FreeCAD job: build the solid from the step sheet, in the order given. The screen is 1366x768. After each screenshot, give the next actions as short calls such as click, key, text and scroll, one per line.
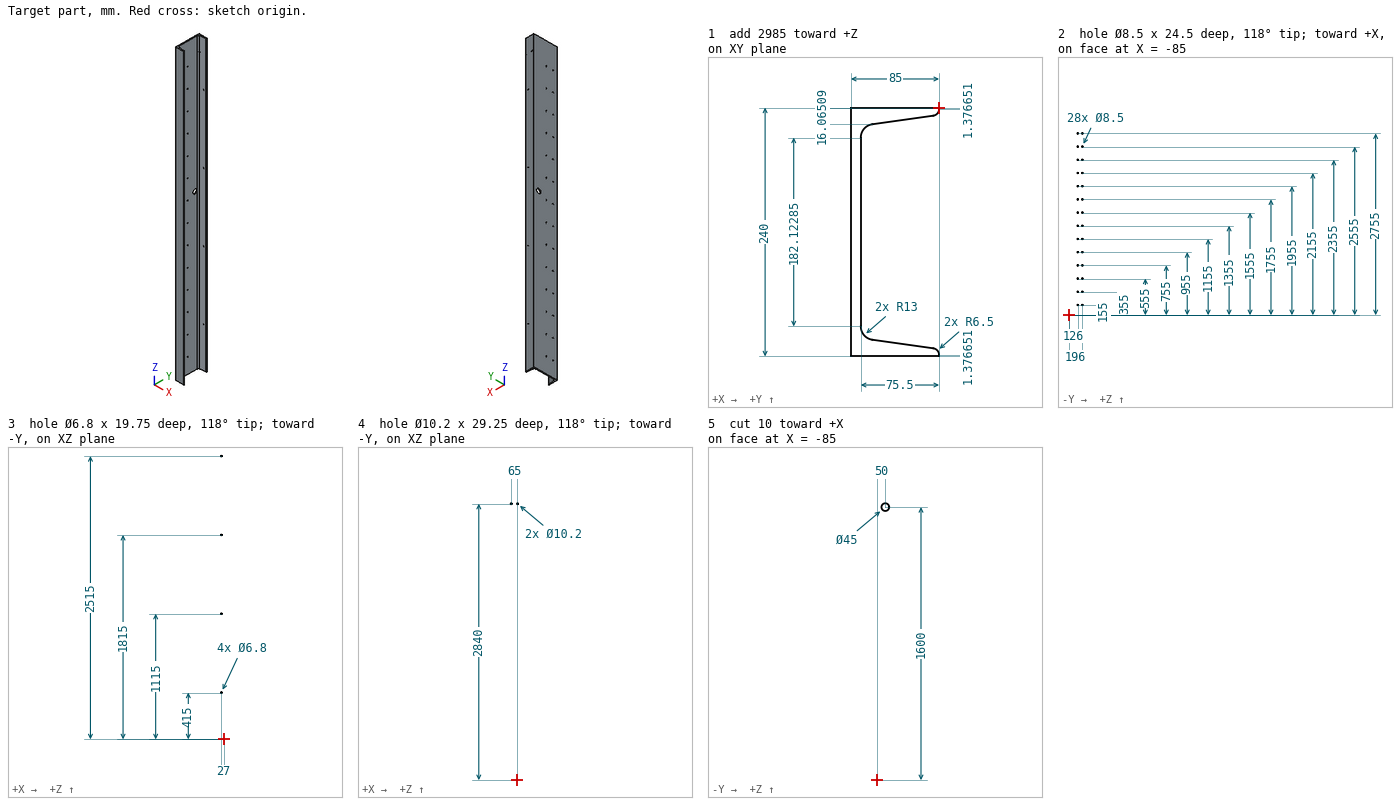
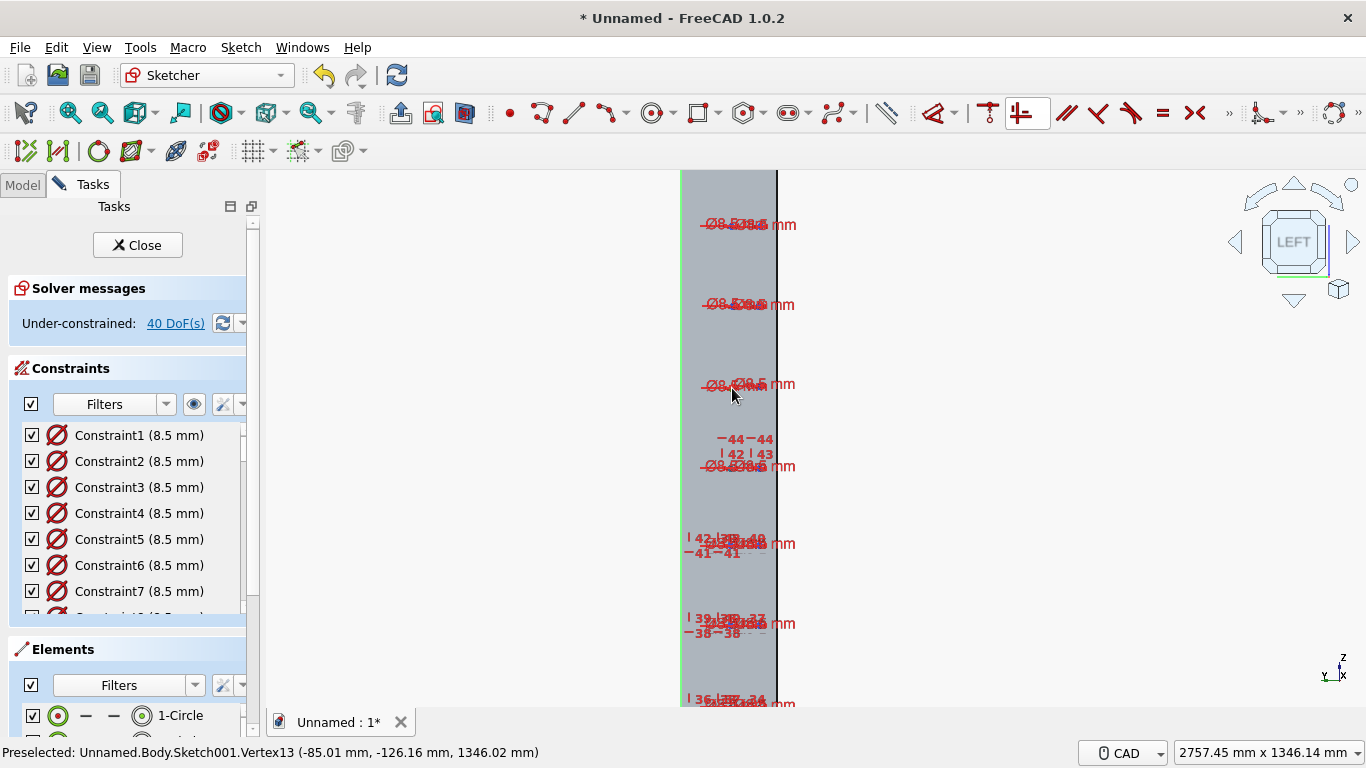
click(1044, 114)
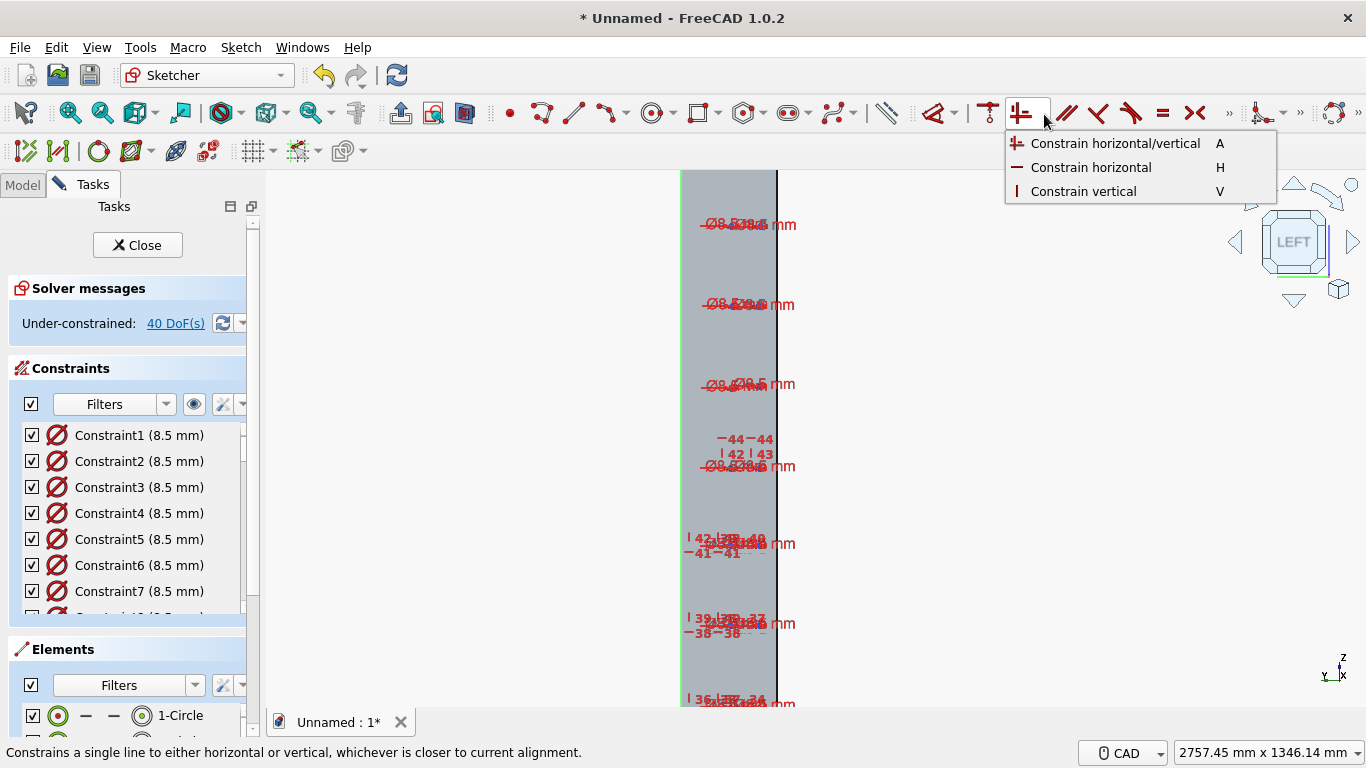
click(1141, 191)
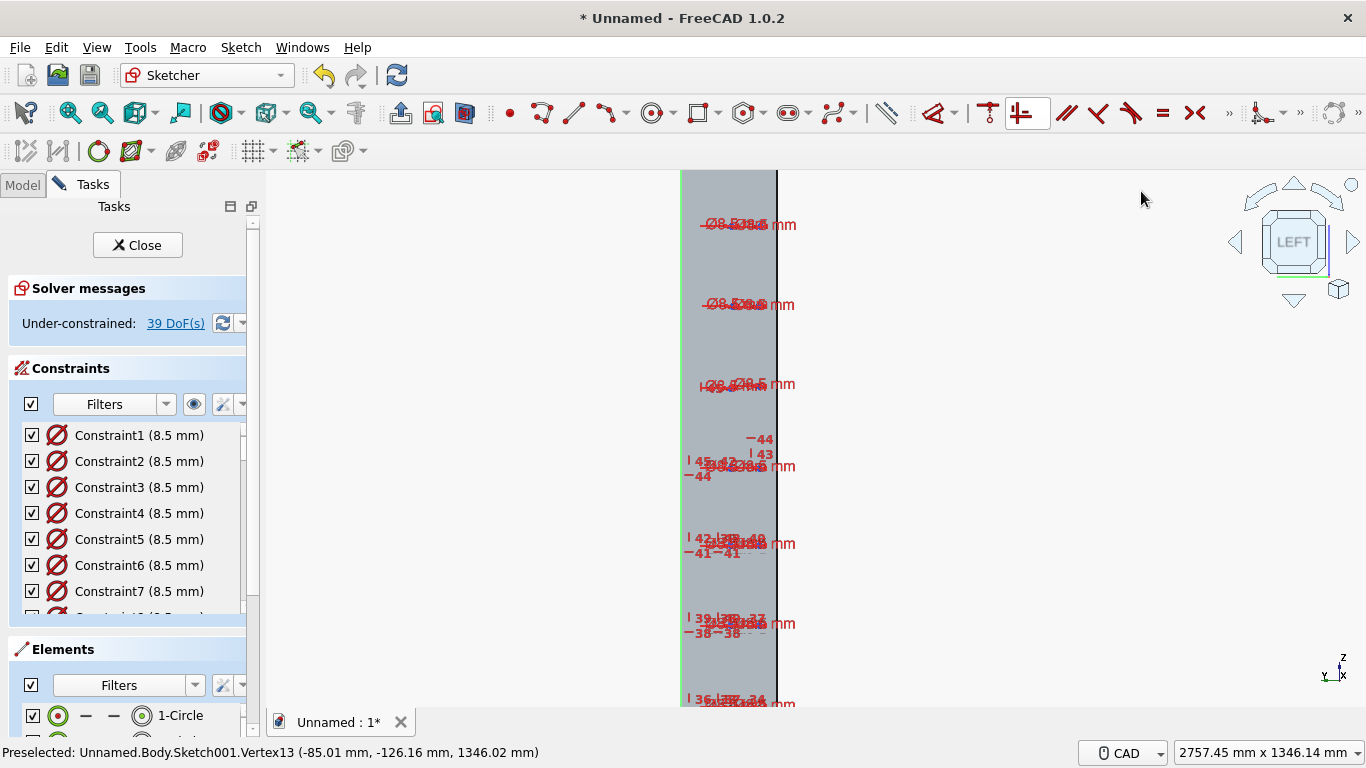
click(759, 468)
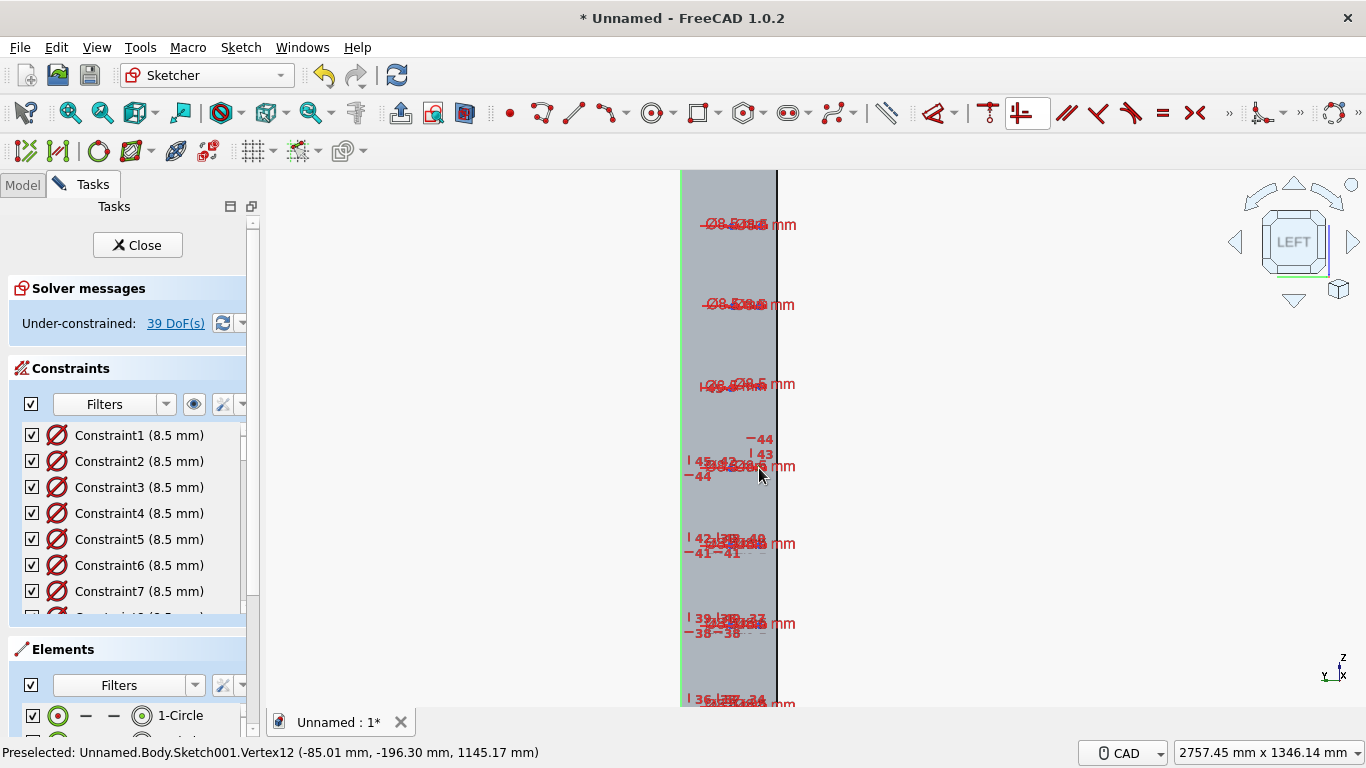
click(759, 386)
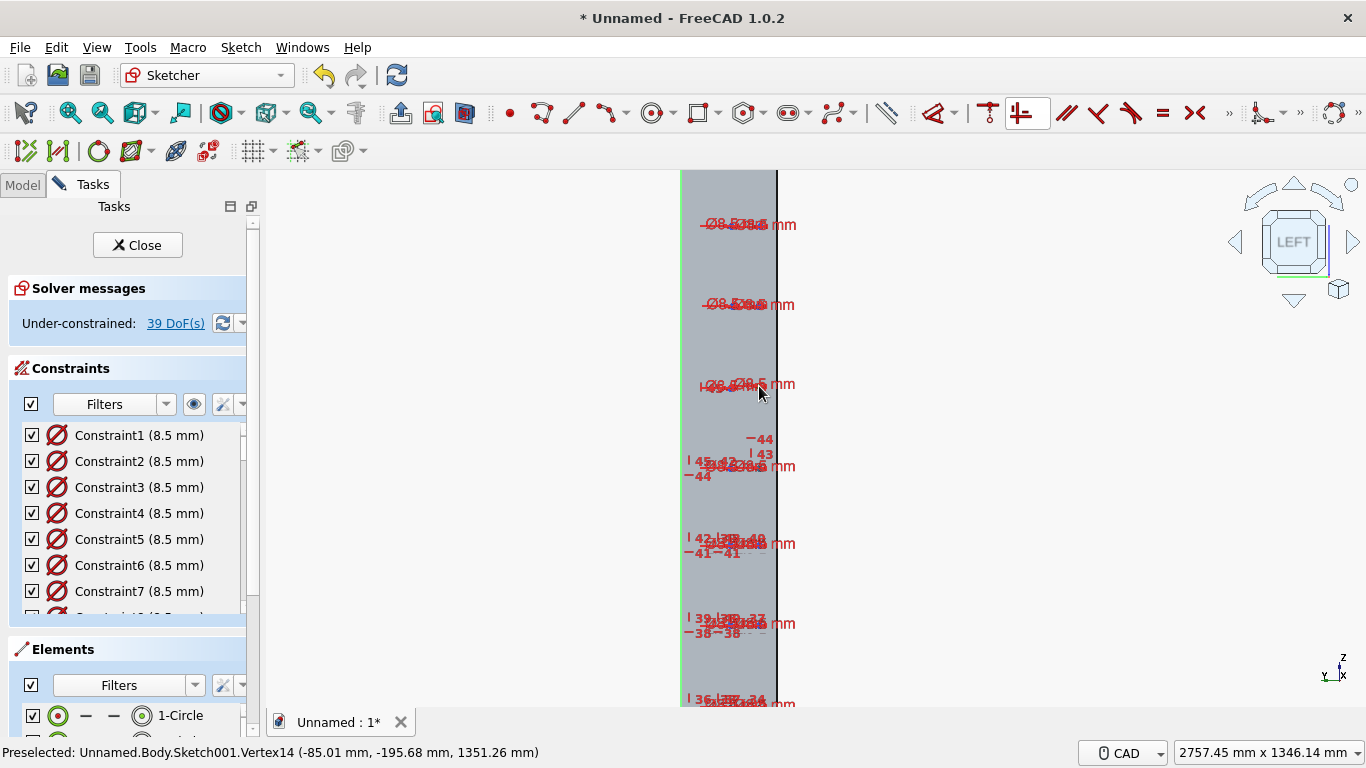
key(v)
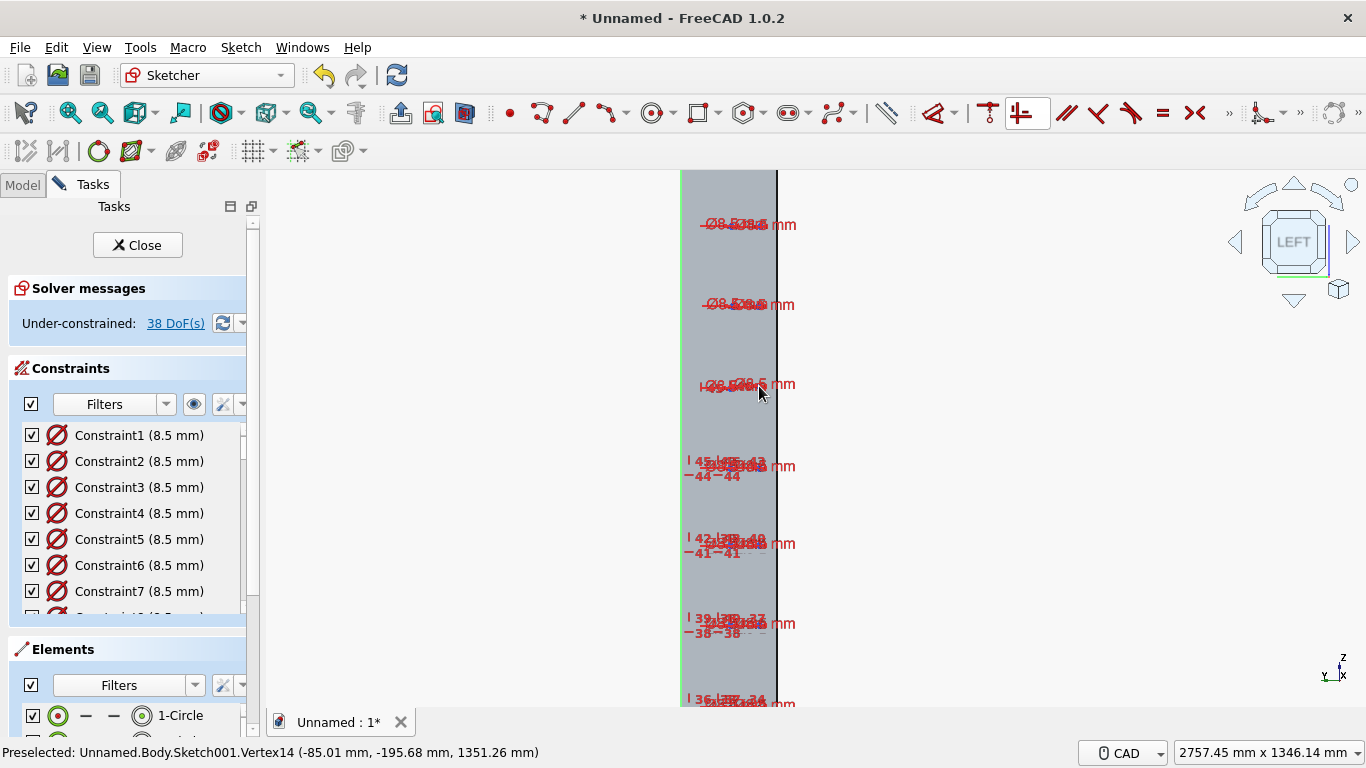
scroll(731, 388, up, 4)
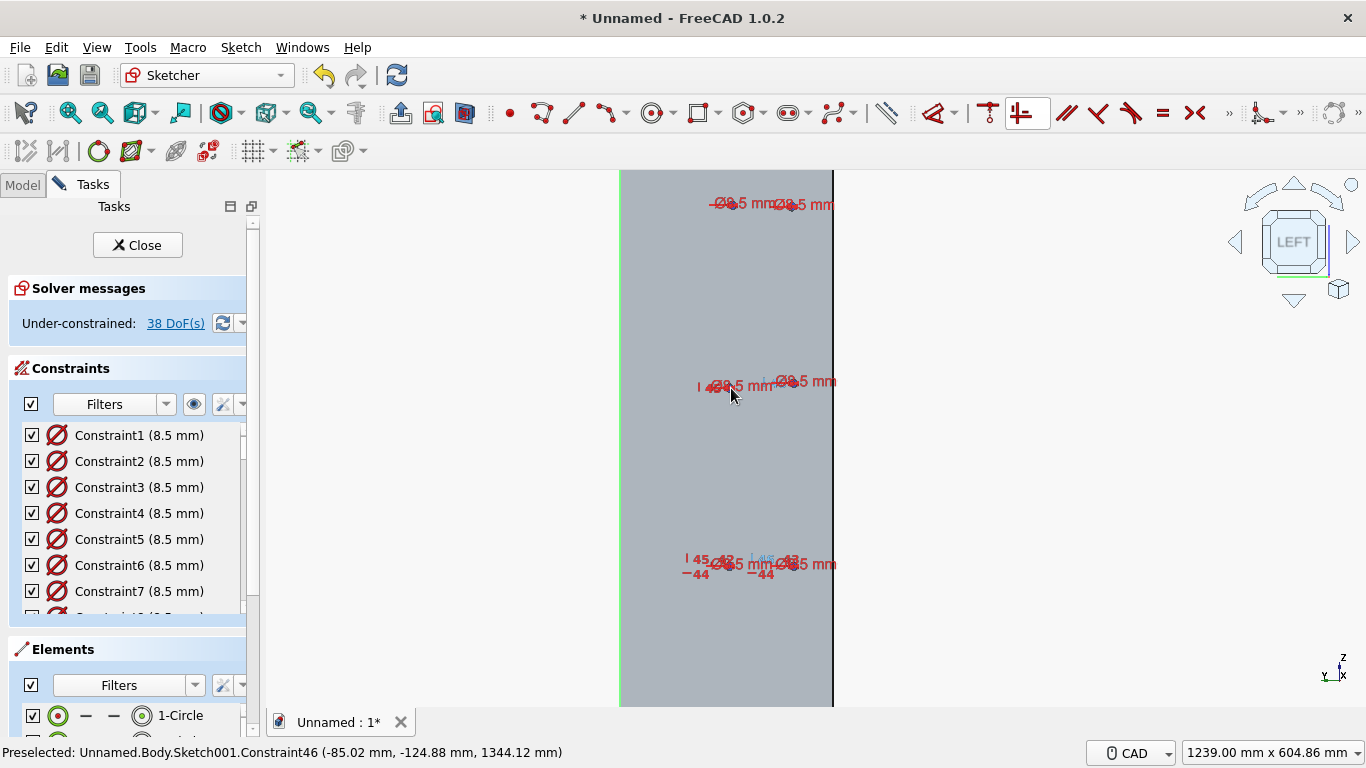
click(729, 388)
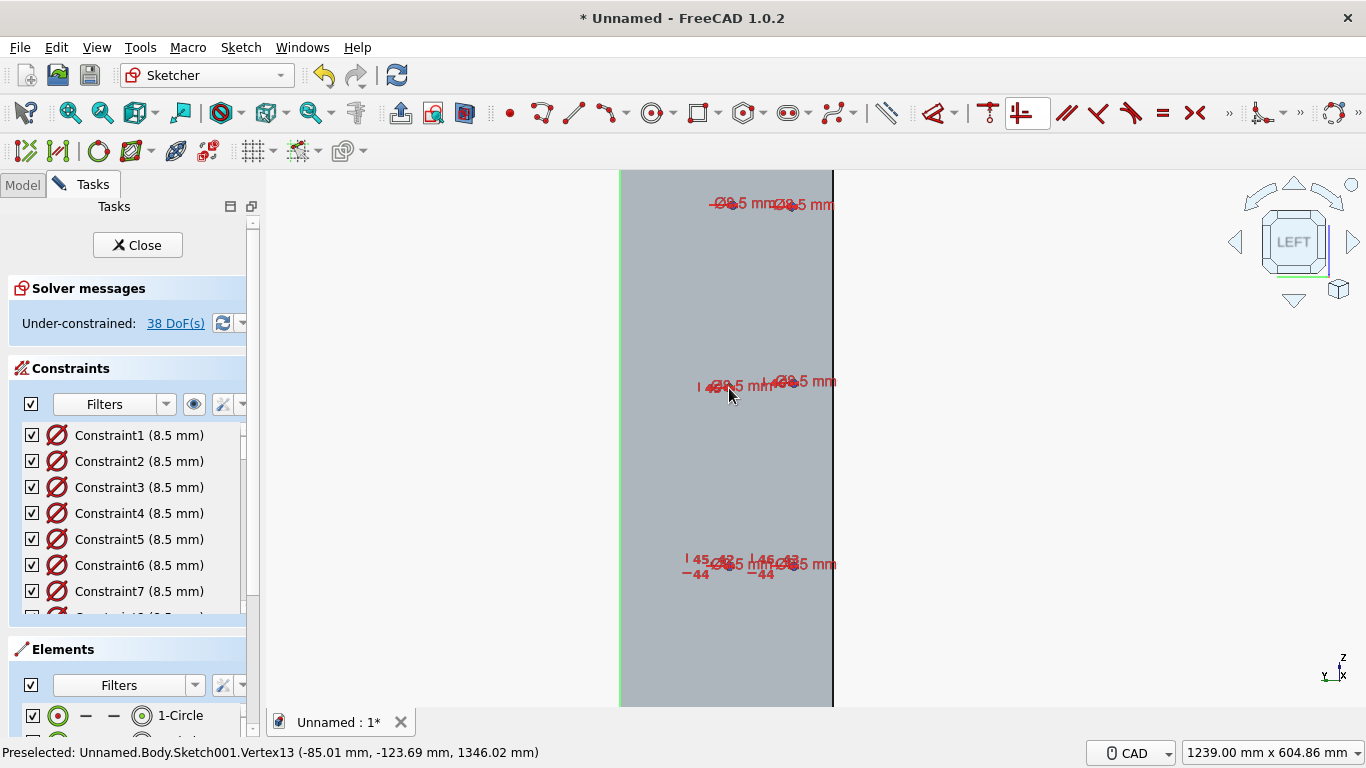
scroll(754, 451, down, 10)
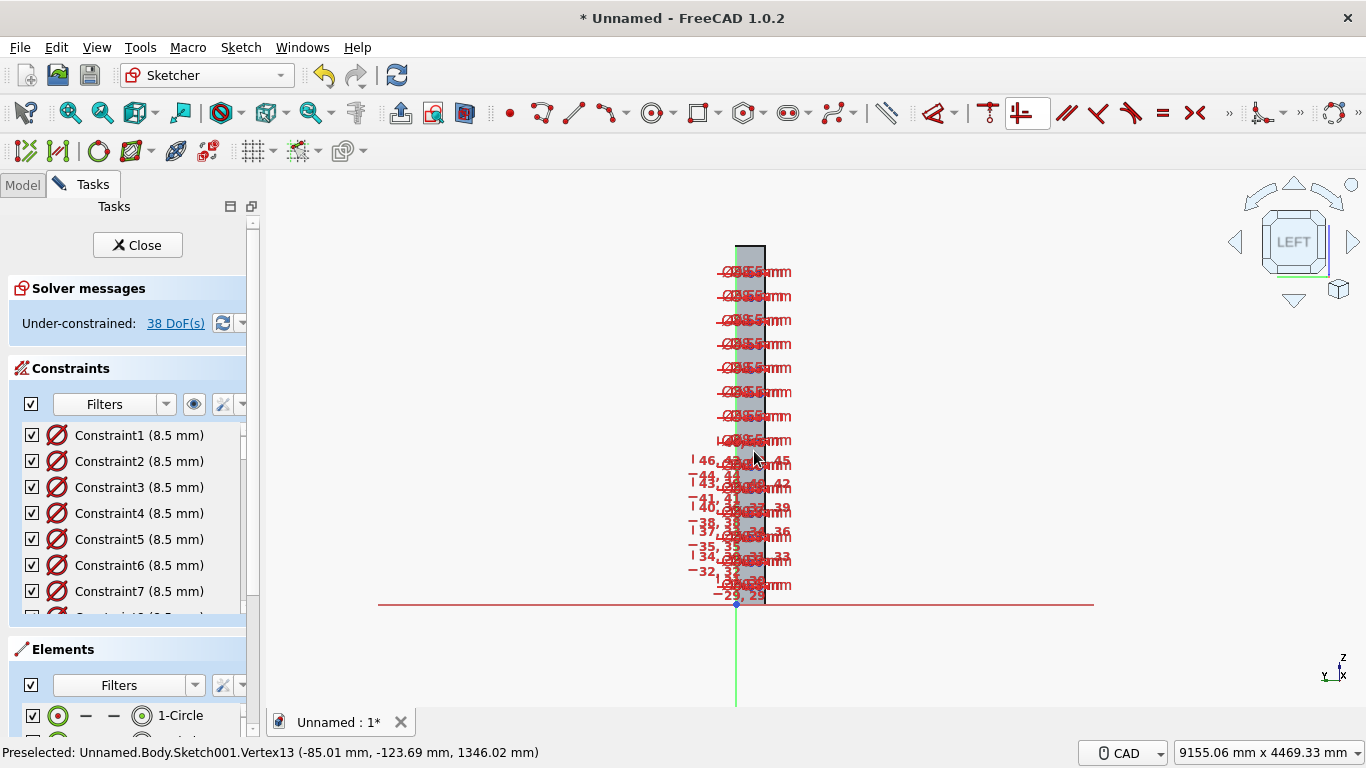
scroll(760, 442, up, 2)